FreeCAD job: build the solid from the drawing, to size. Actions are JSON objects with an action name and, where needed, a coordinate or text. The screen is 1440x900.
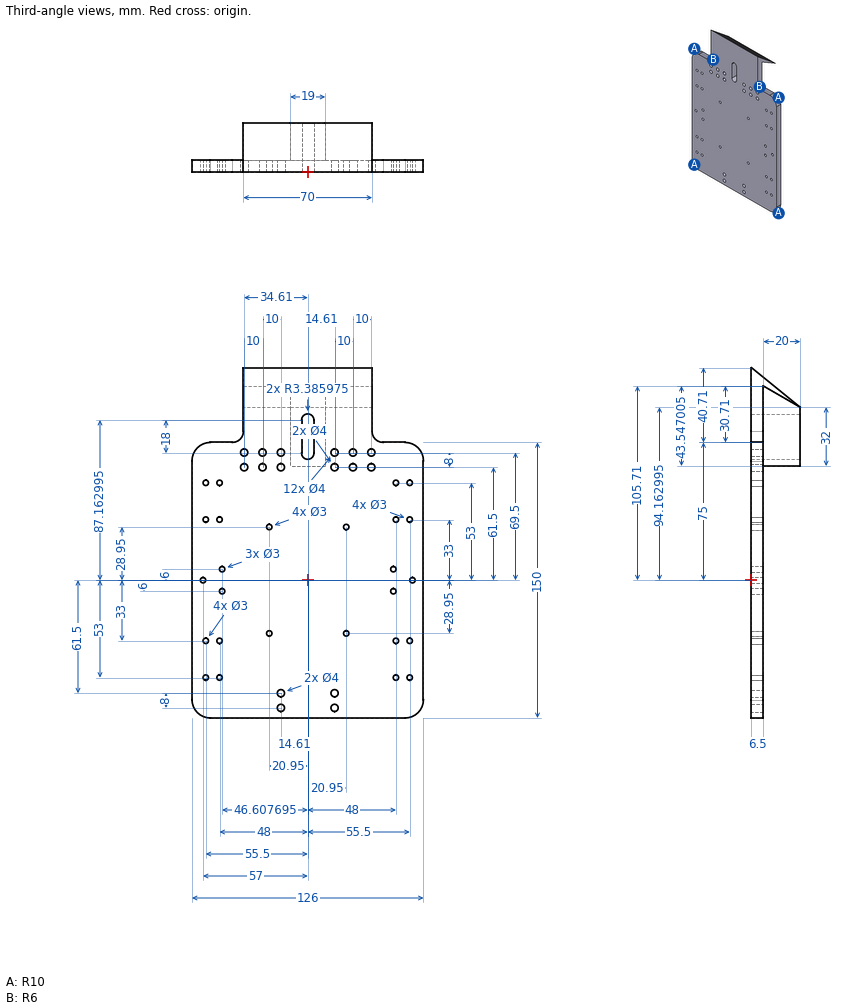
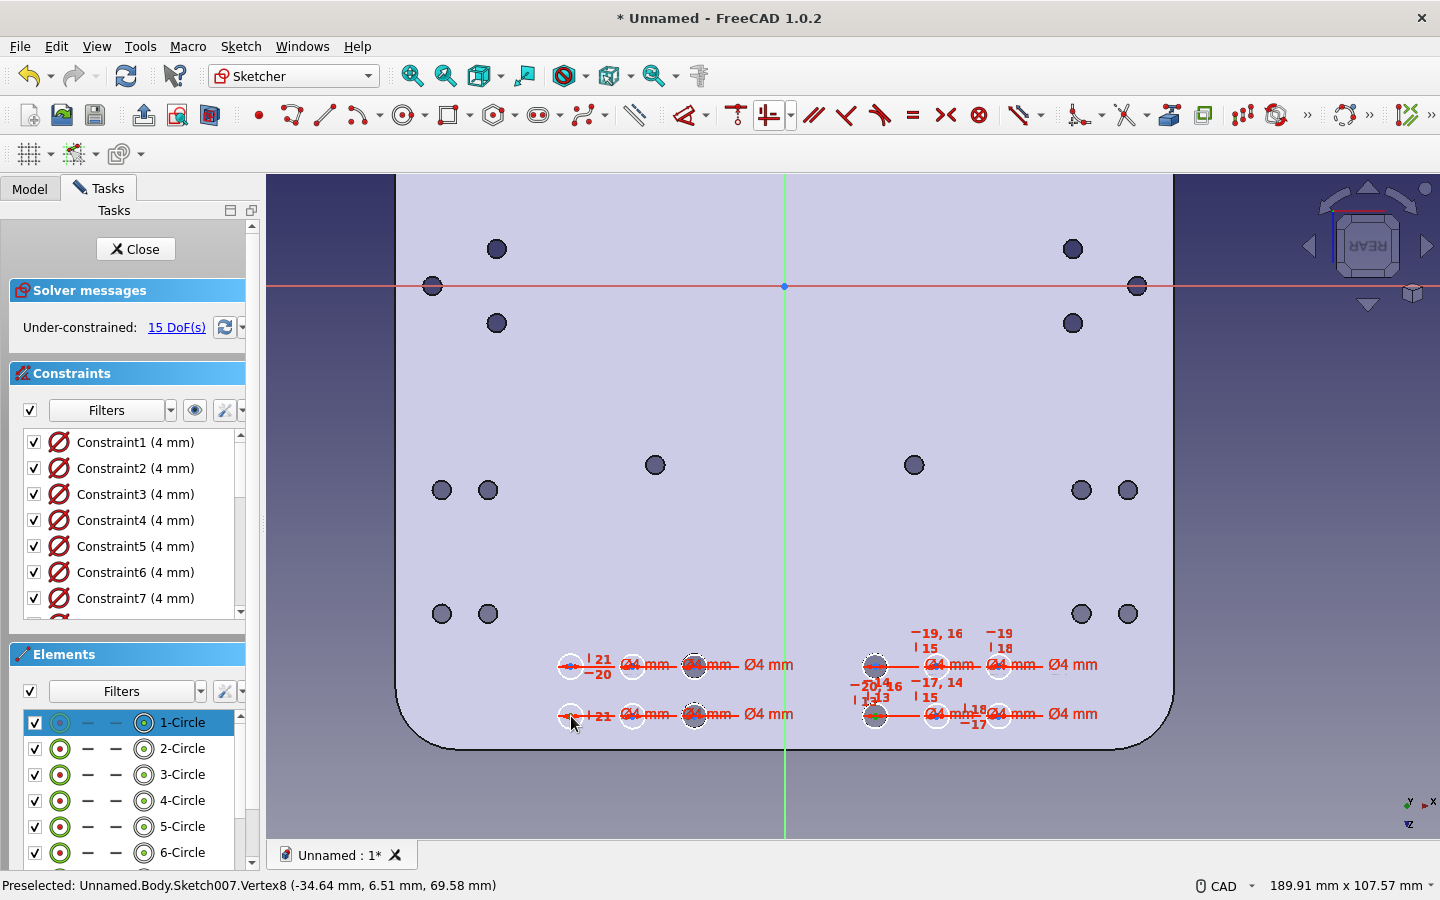
{"action": "left_click", "coordinate": [790, 116]}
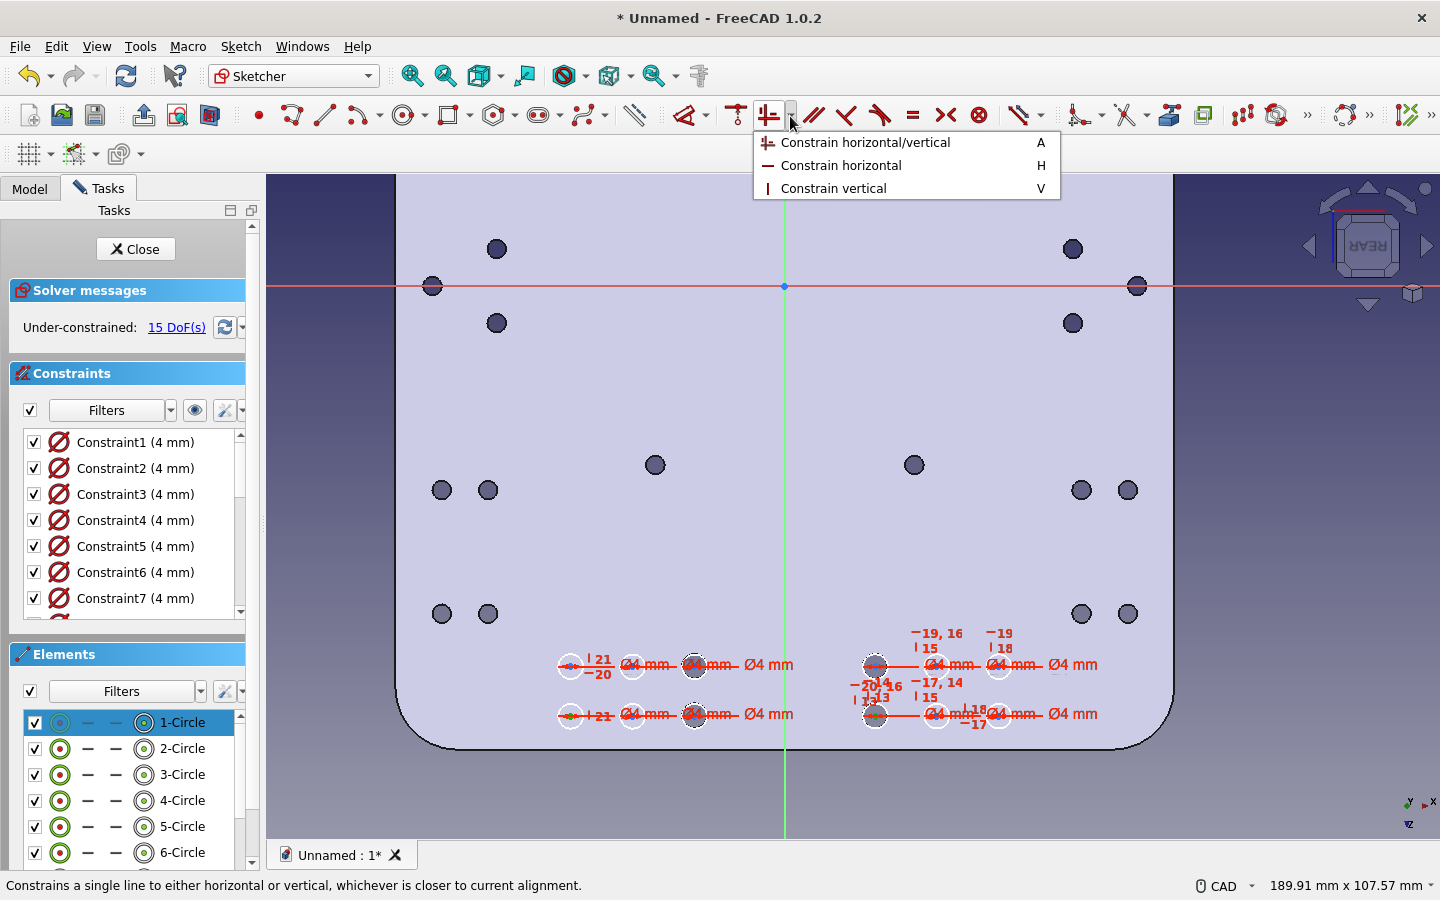
{"action": "left_click", "coordinate": [907, 166]}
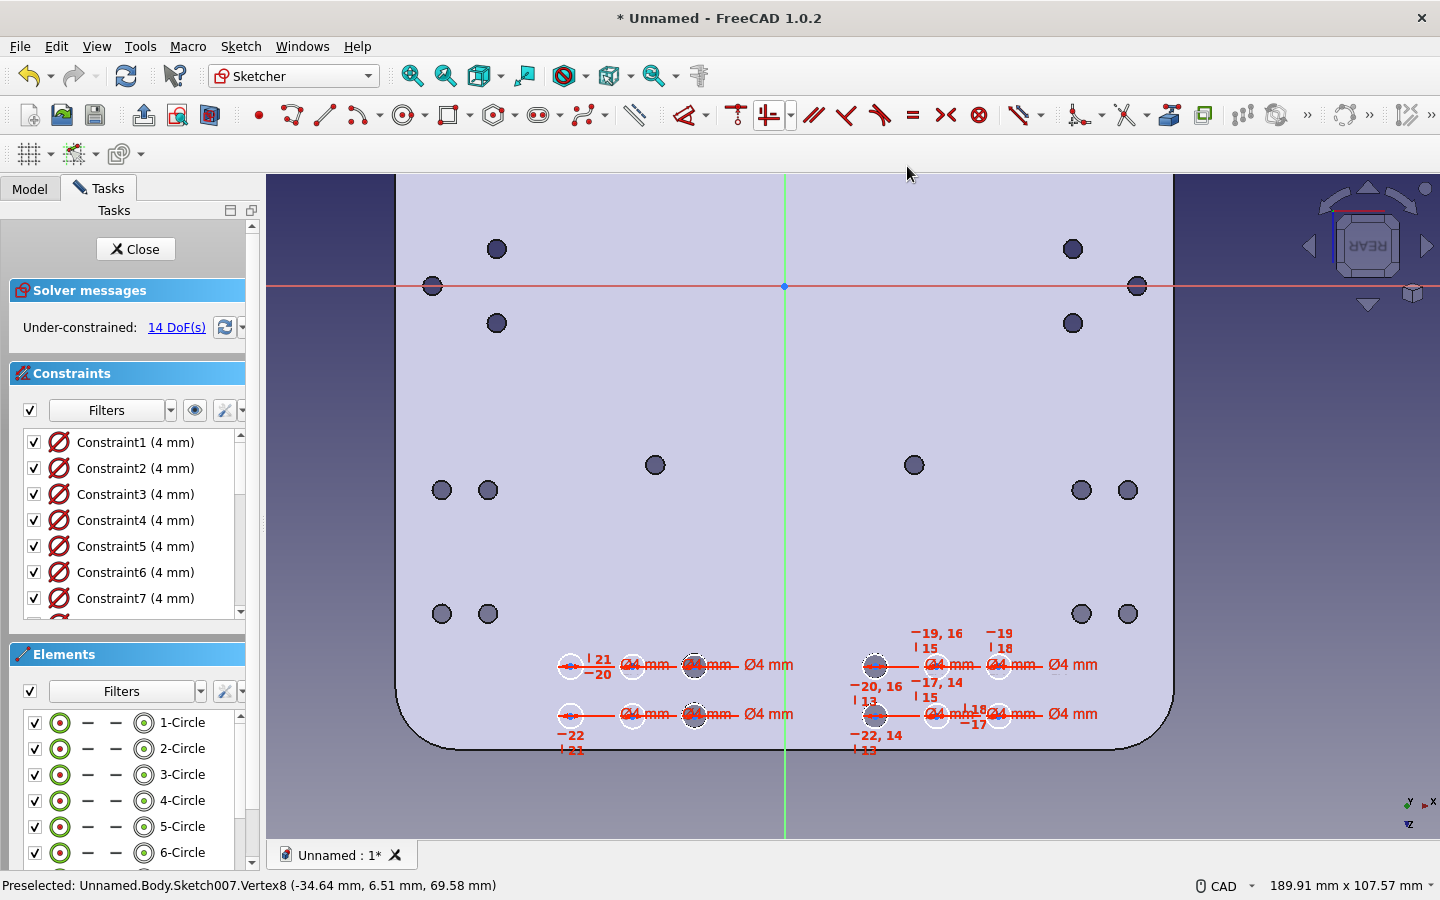
{"action": "left_click", "coordinate": [571, 667]}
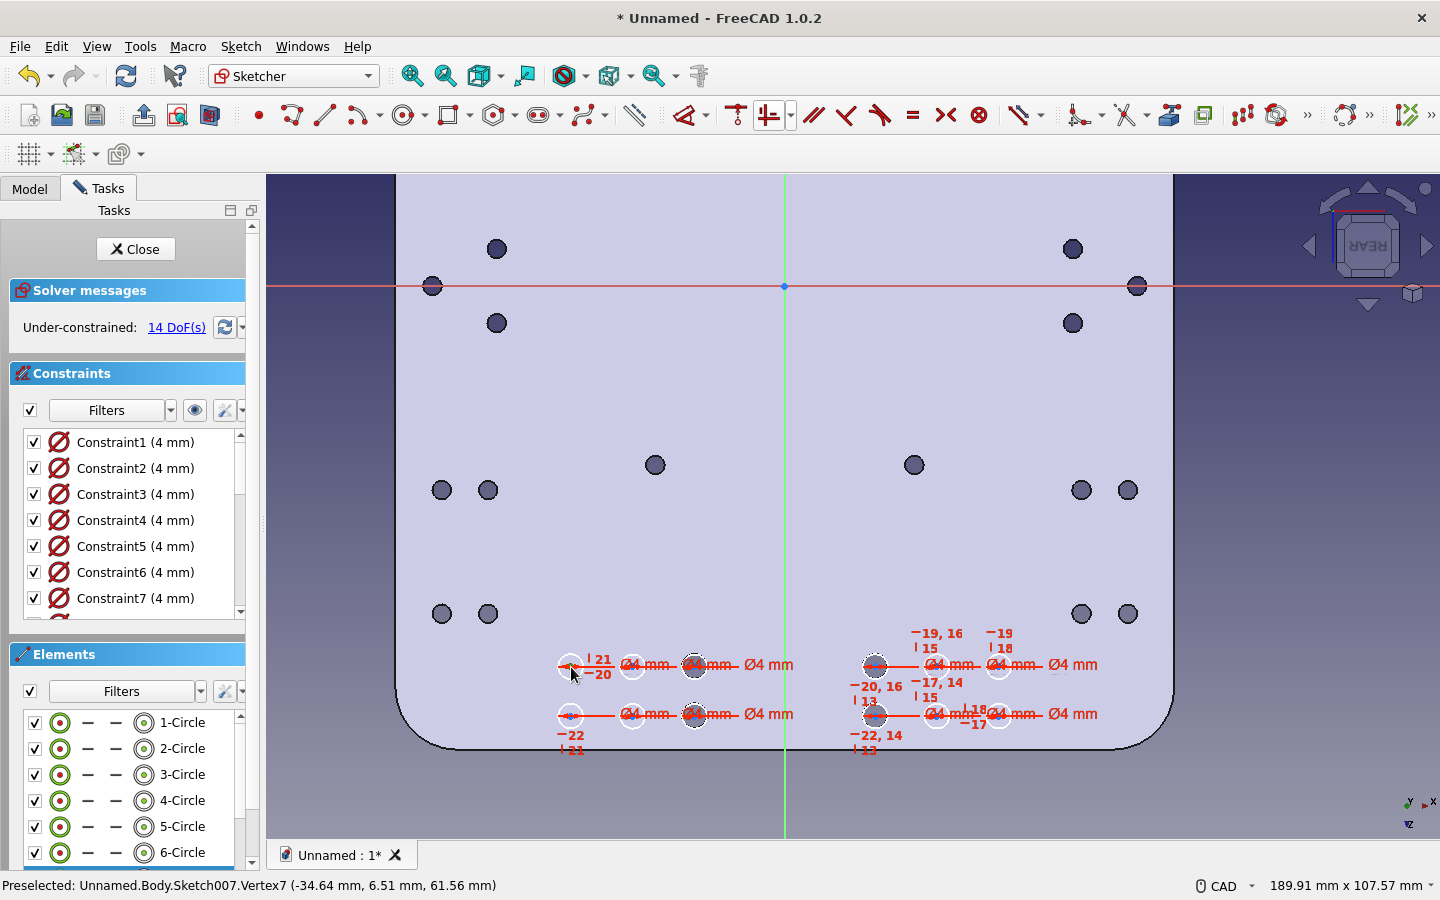
{"action": "left_click", "coordinate": [633, 667]}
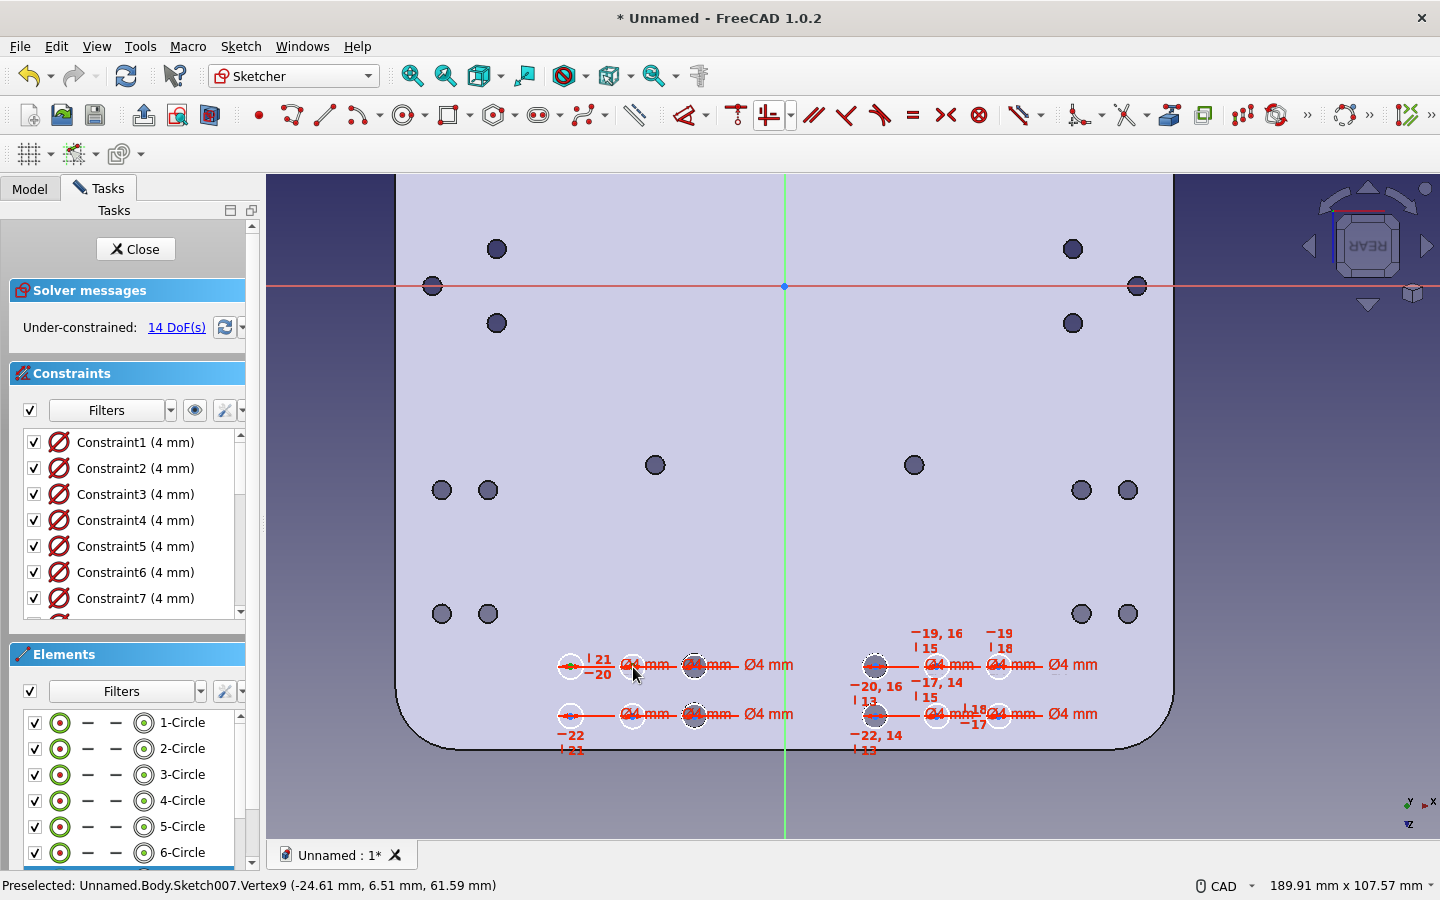
{"action": "key", "text": "h"}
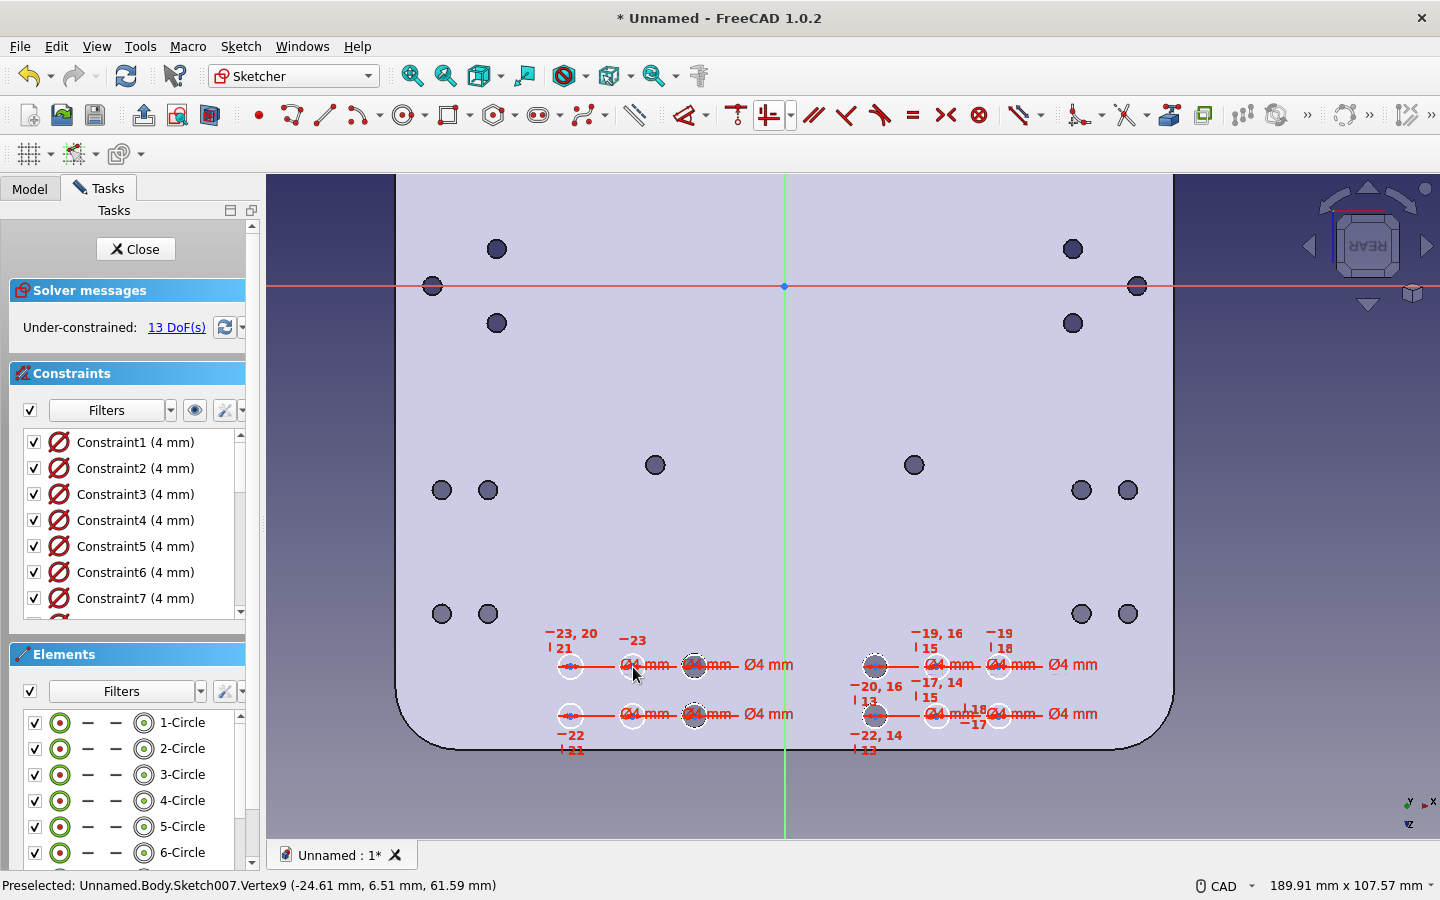
{"action": "left_click", "coordinate": [633, 667]}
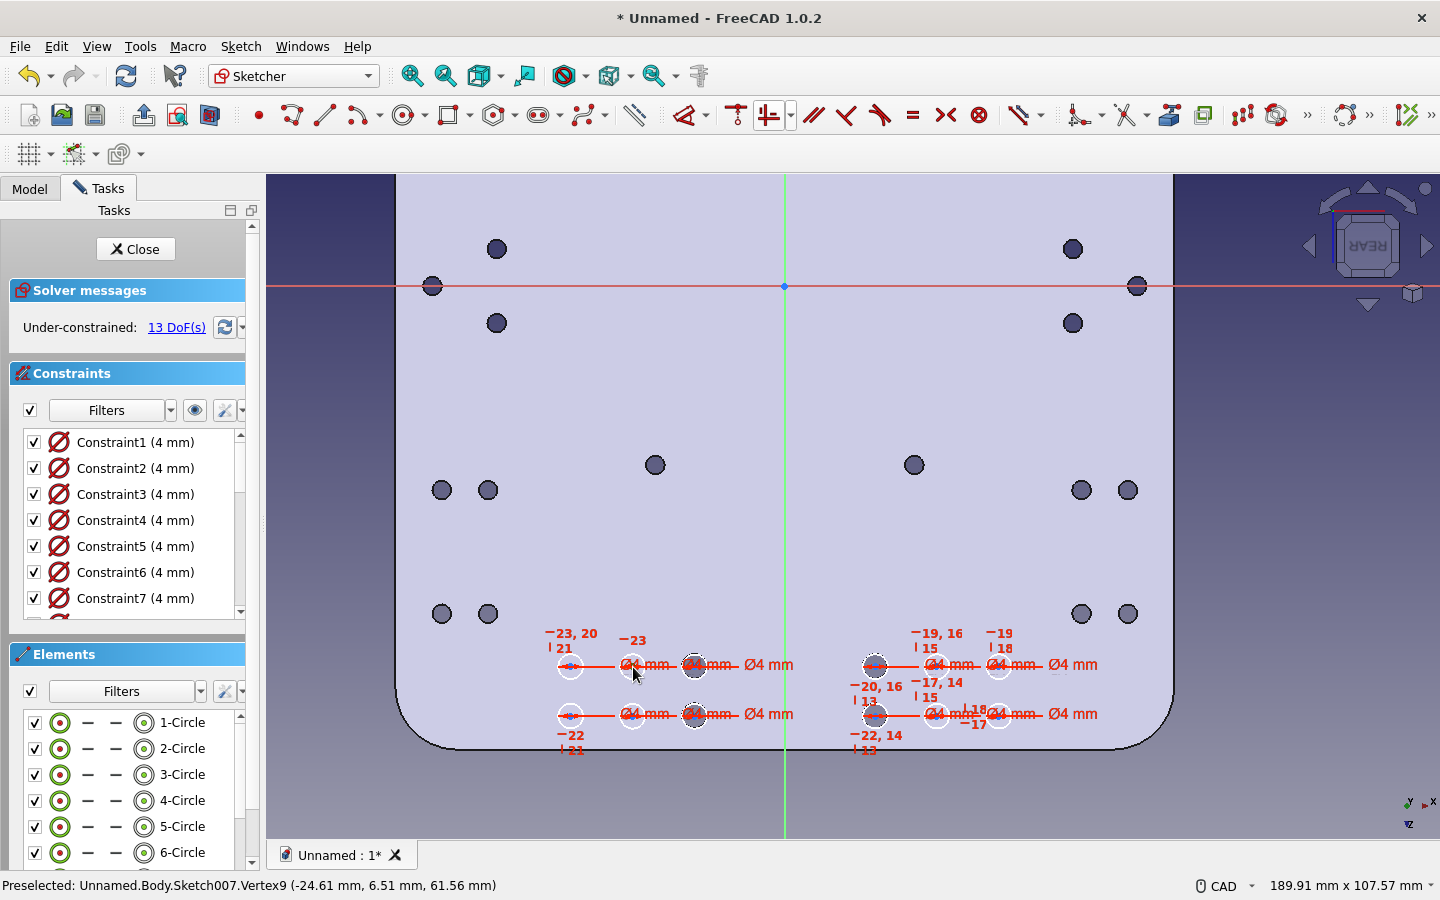
{"action": "left_click", "coordinate": [633, 716]}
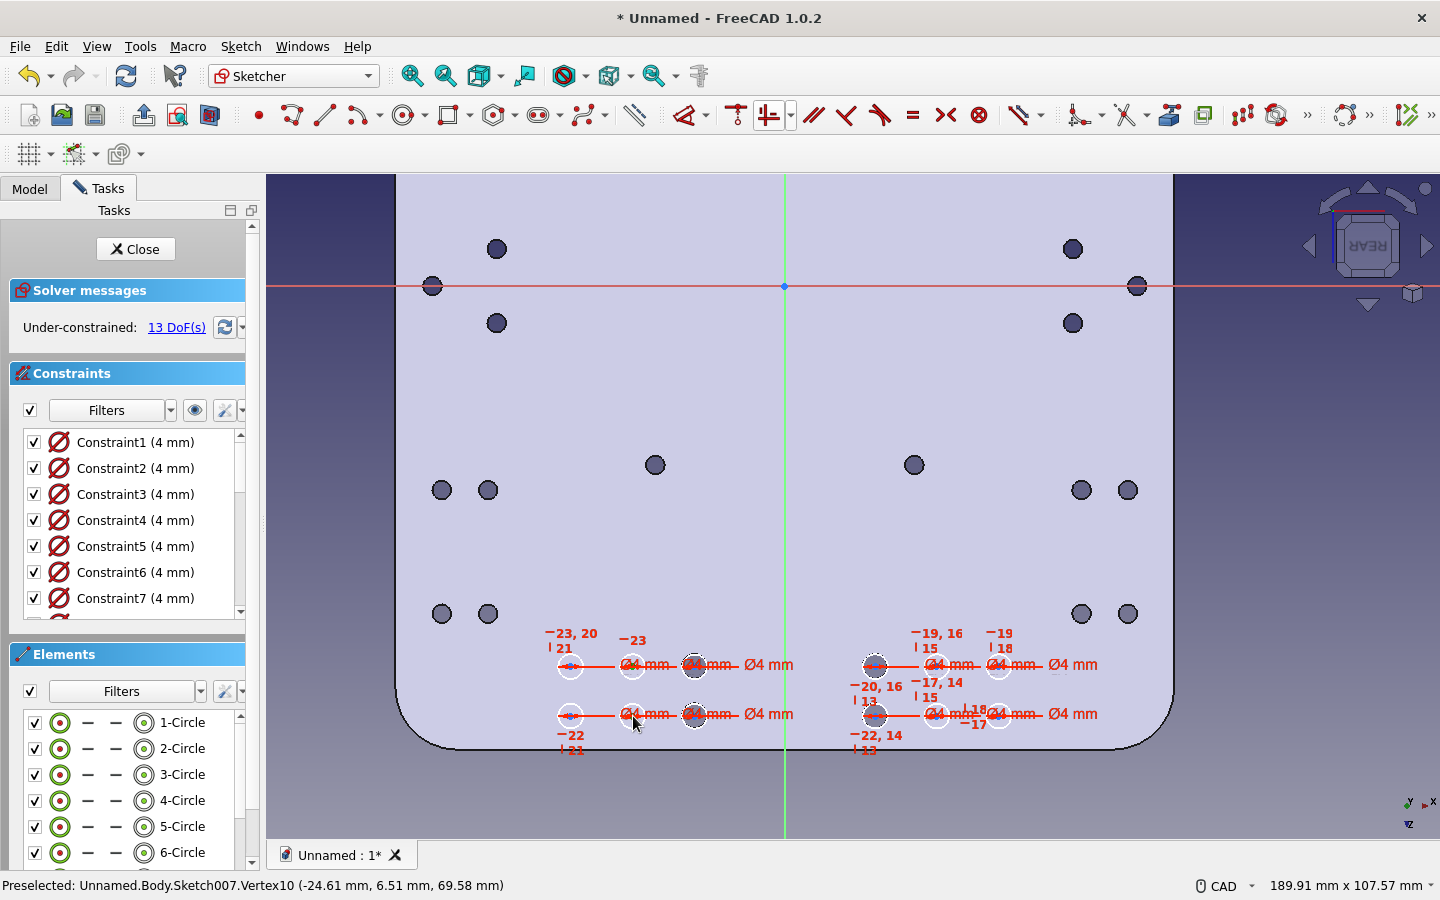
{"action": "left_click", "coordinate": [790, 116]}